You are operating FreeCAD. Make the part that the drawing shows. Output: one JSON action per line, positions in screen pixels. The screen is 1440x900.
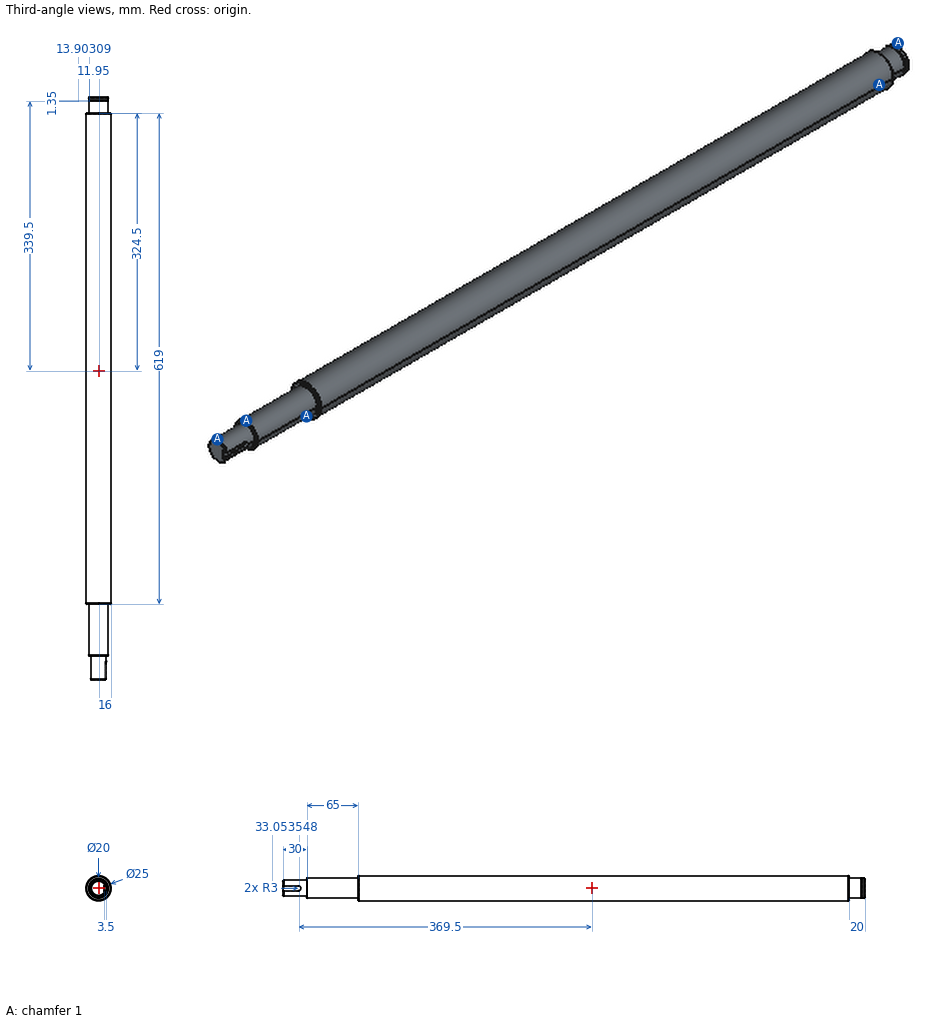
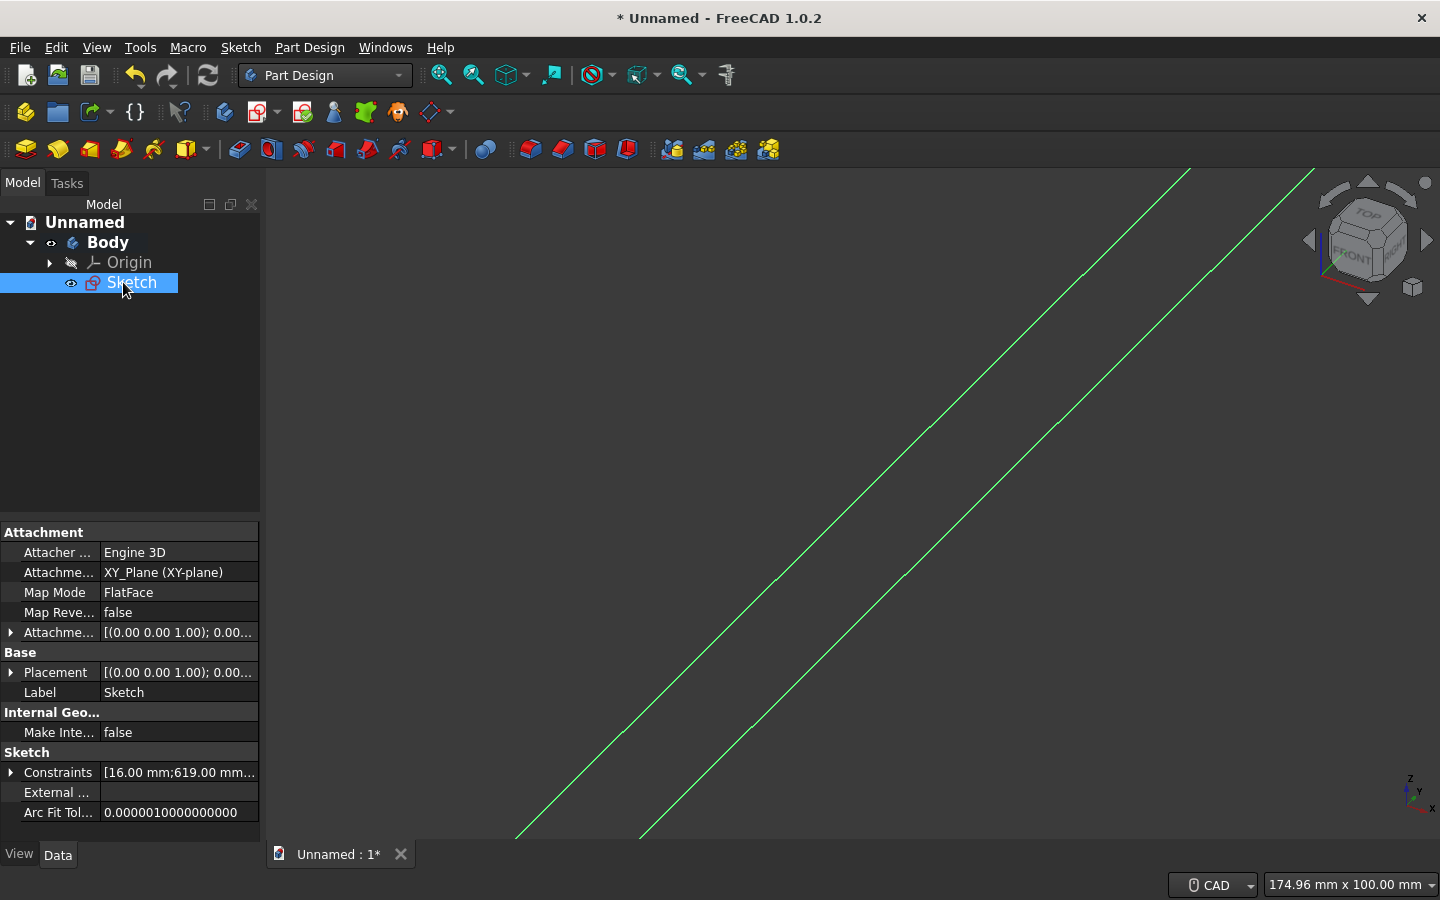
{"action": "left_click", "coordinate": [58, 150]}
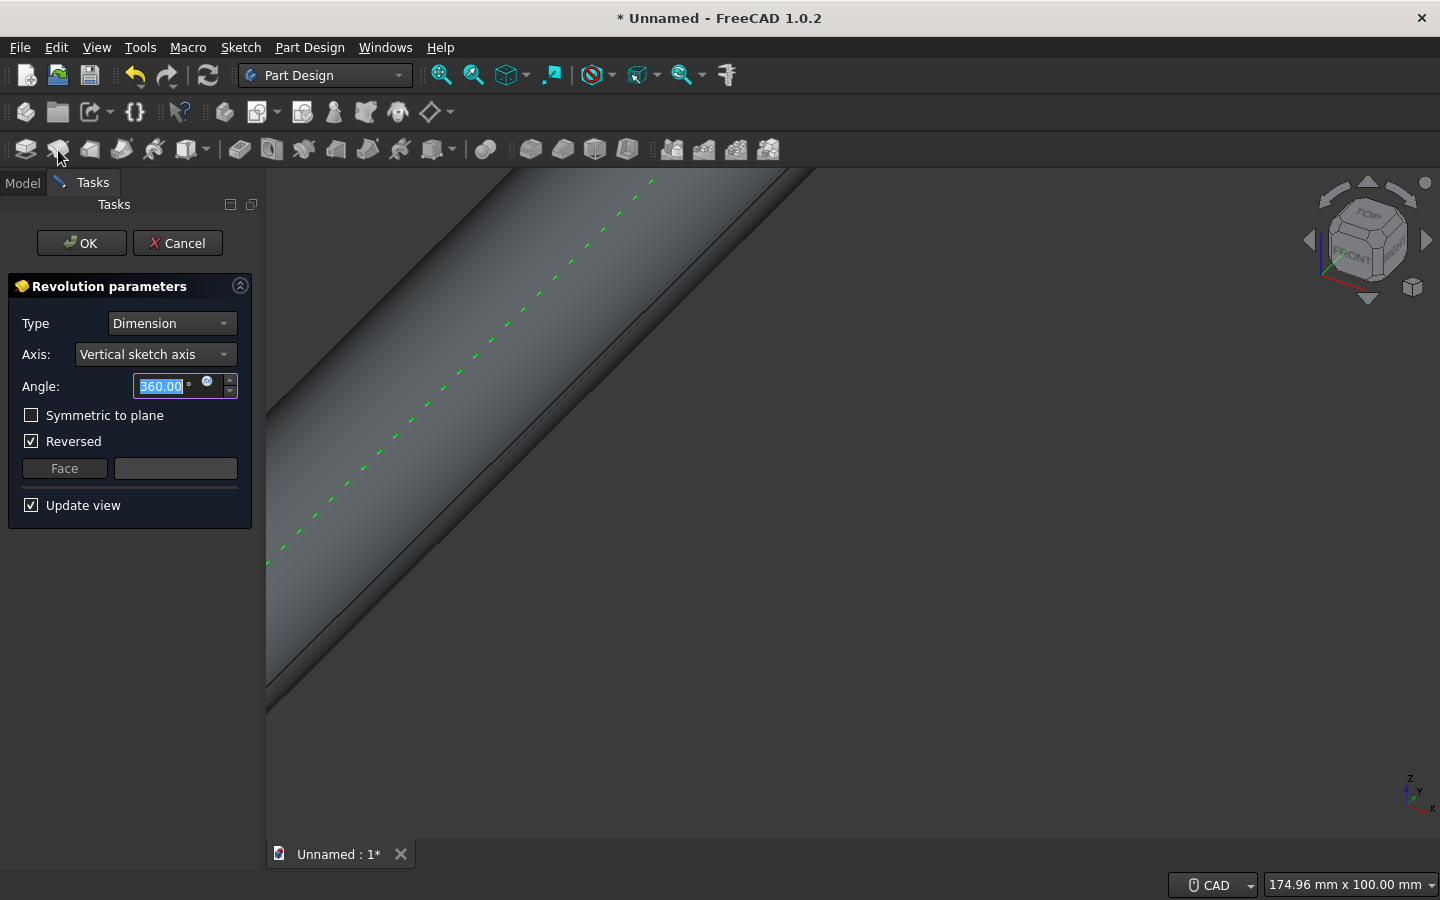
{"action": "left_click", "coordinate": [82, 243]}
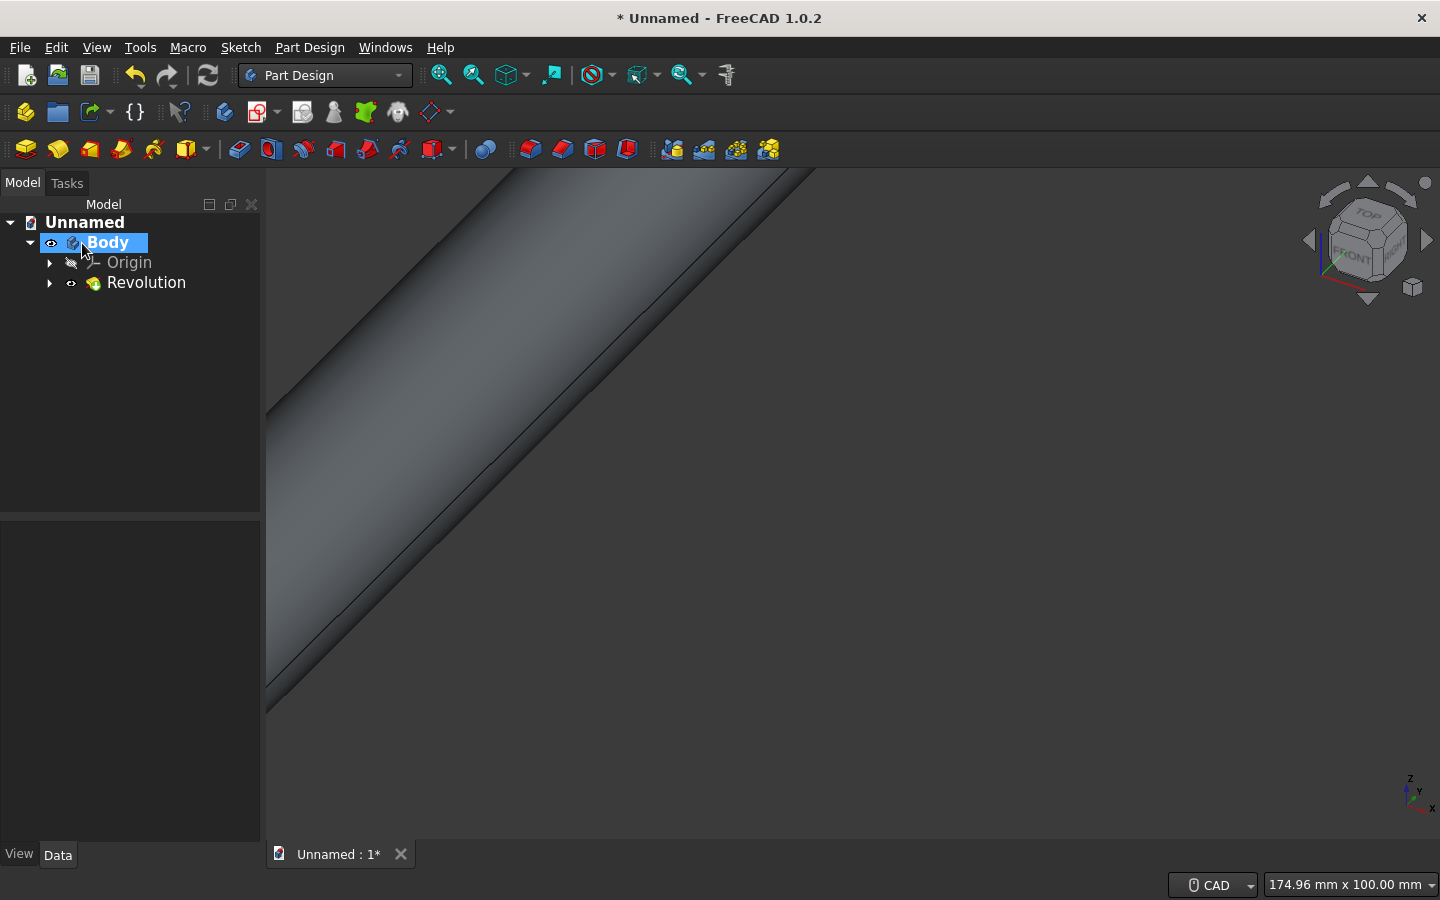
{"action": "left_click", "coordinate": [442, 76]}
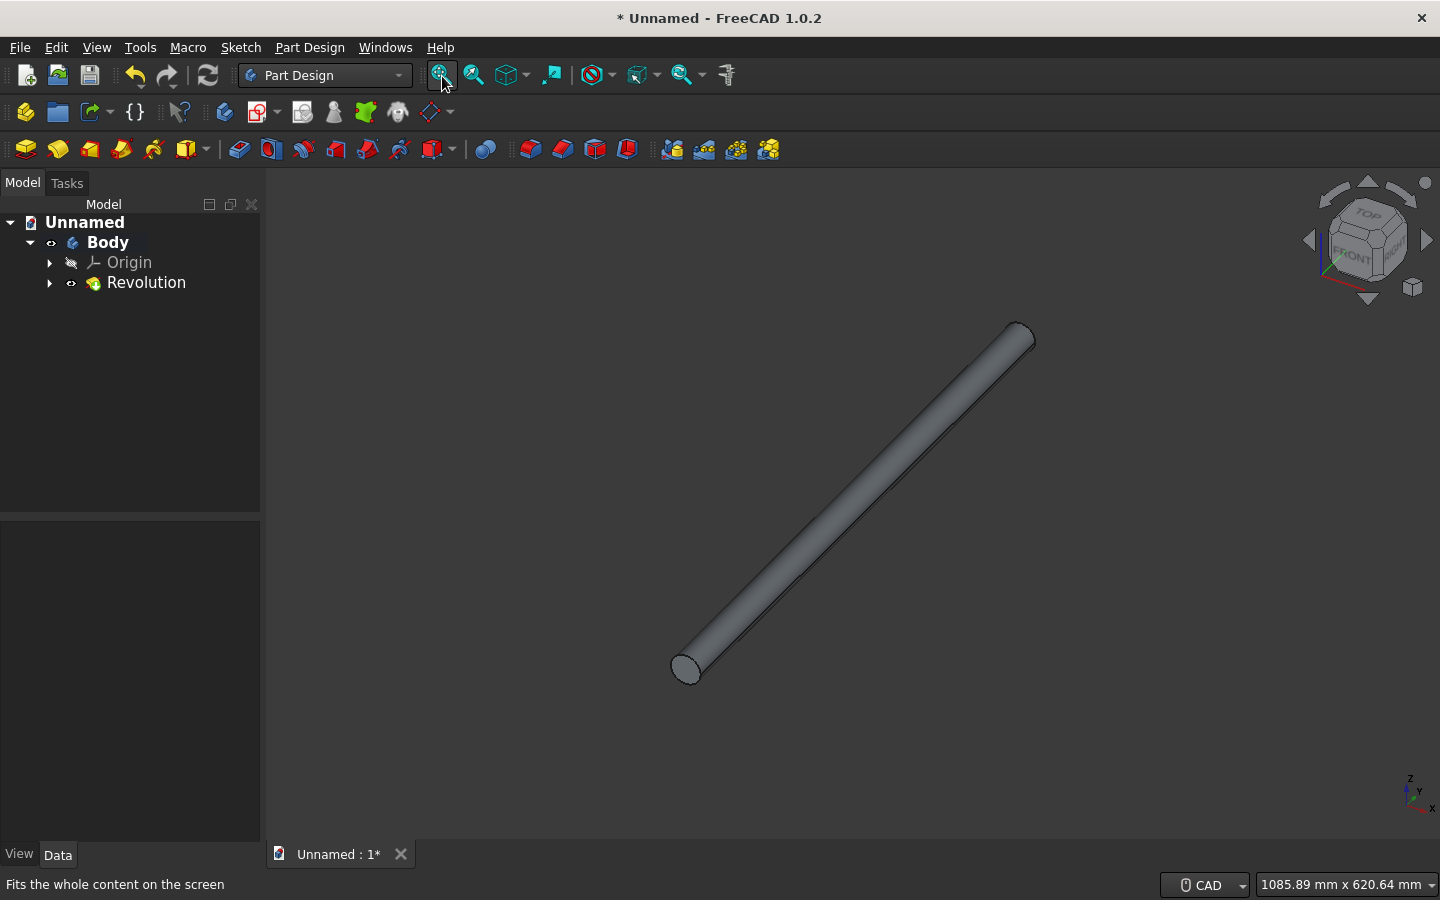
{"action": "left_click", "coordinate": [686, 669]}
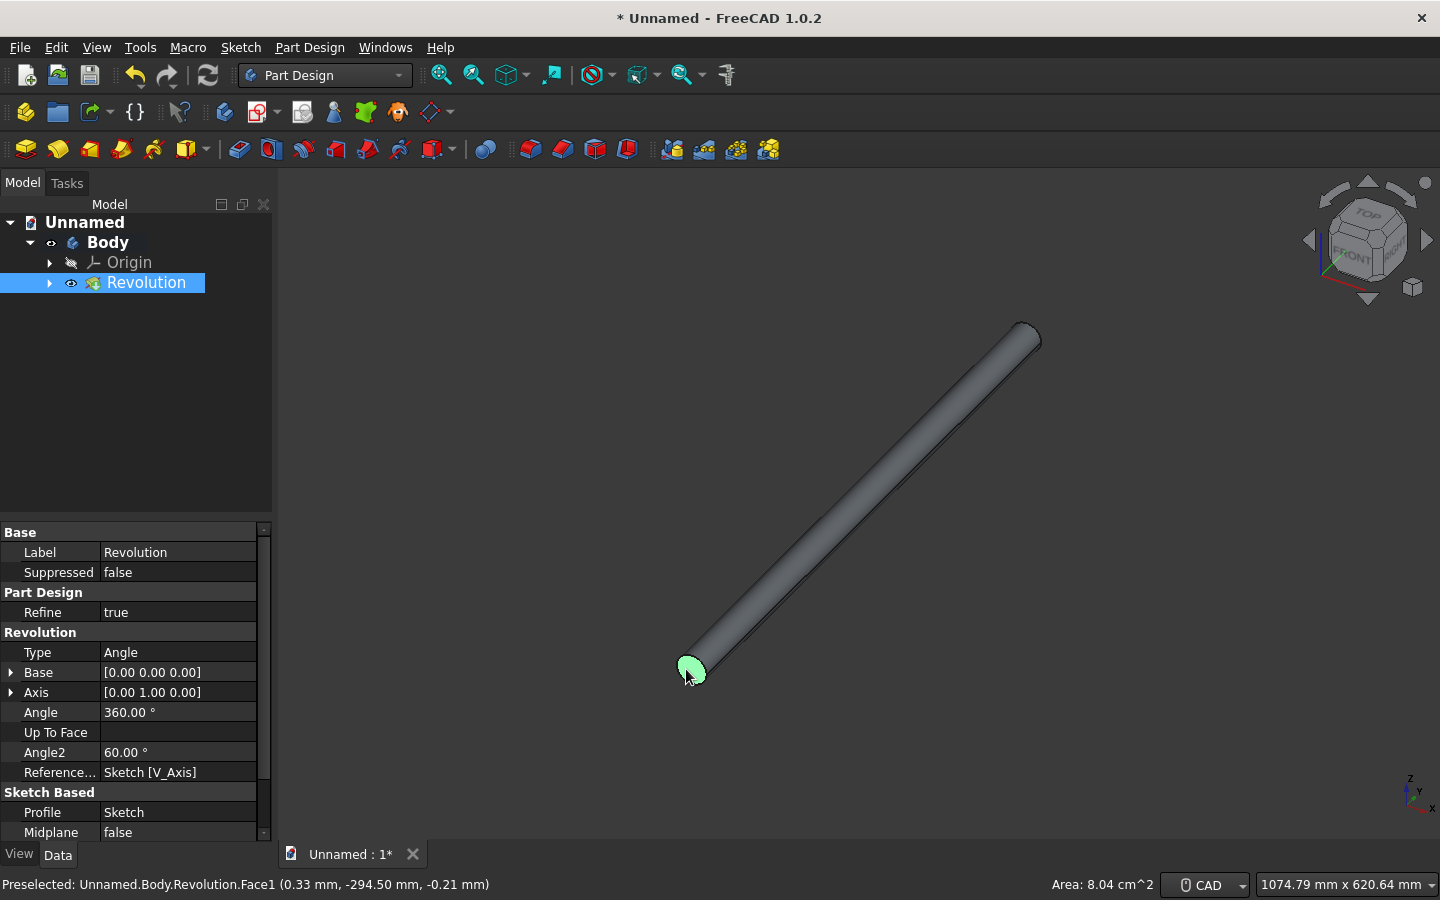
{"action": "left_click", "coordinate": [258, 112]}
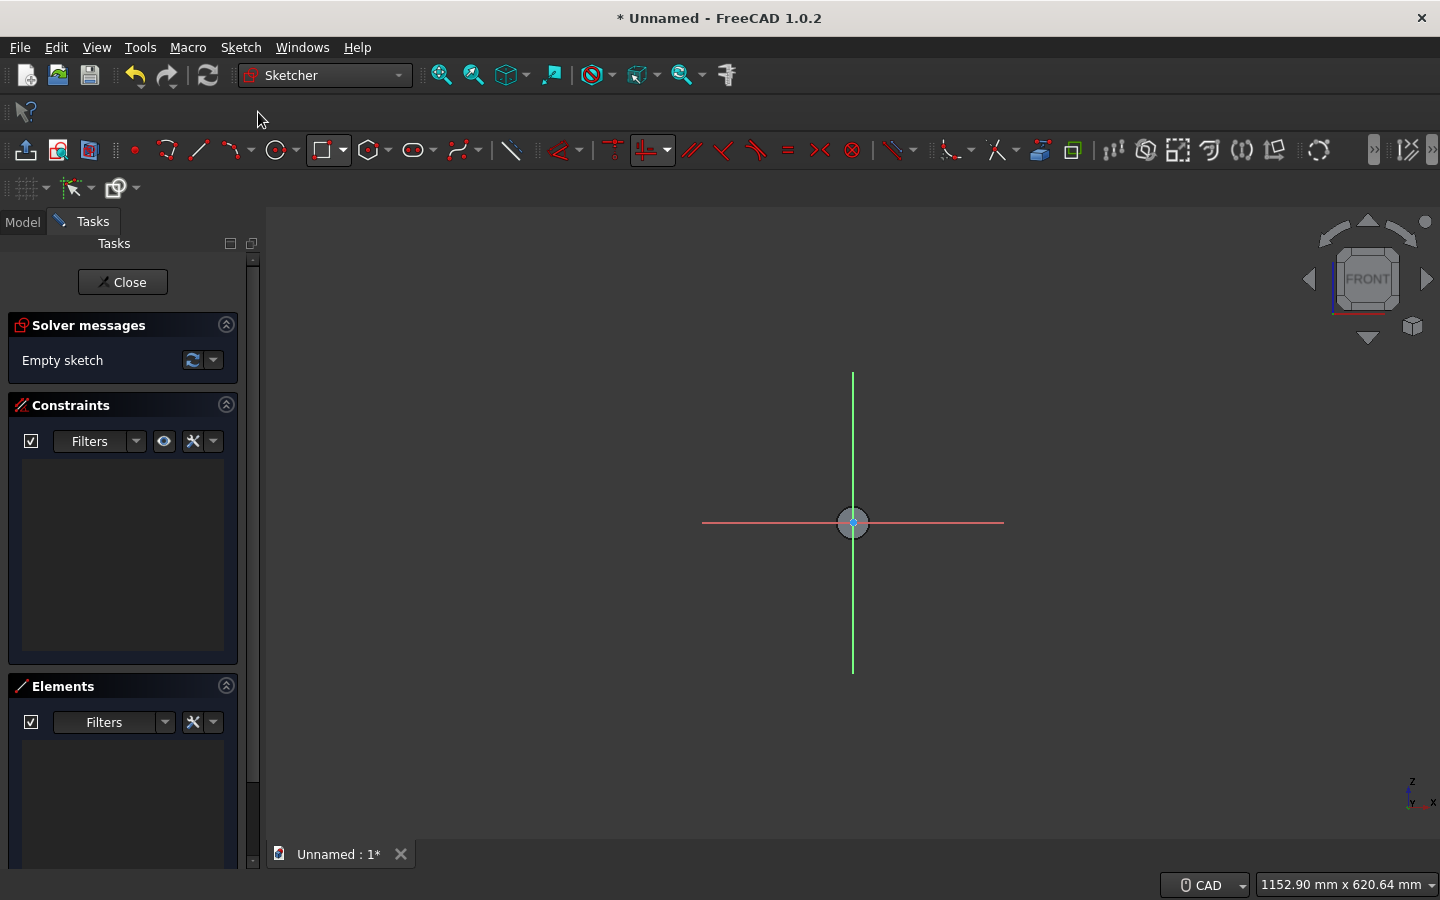
{"action": "scroll", "coordinate": [857, 523], "scroll_direction": "up", "scroll_amount": 14}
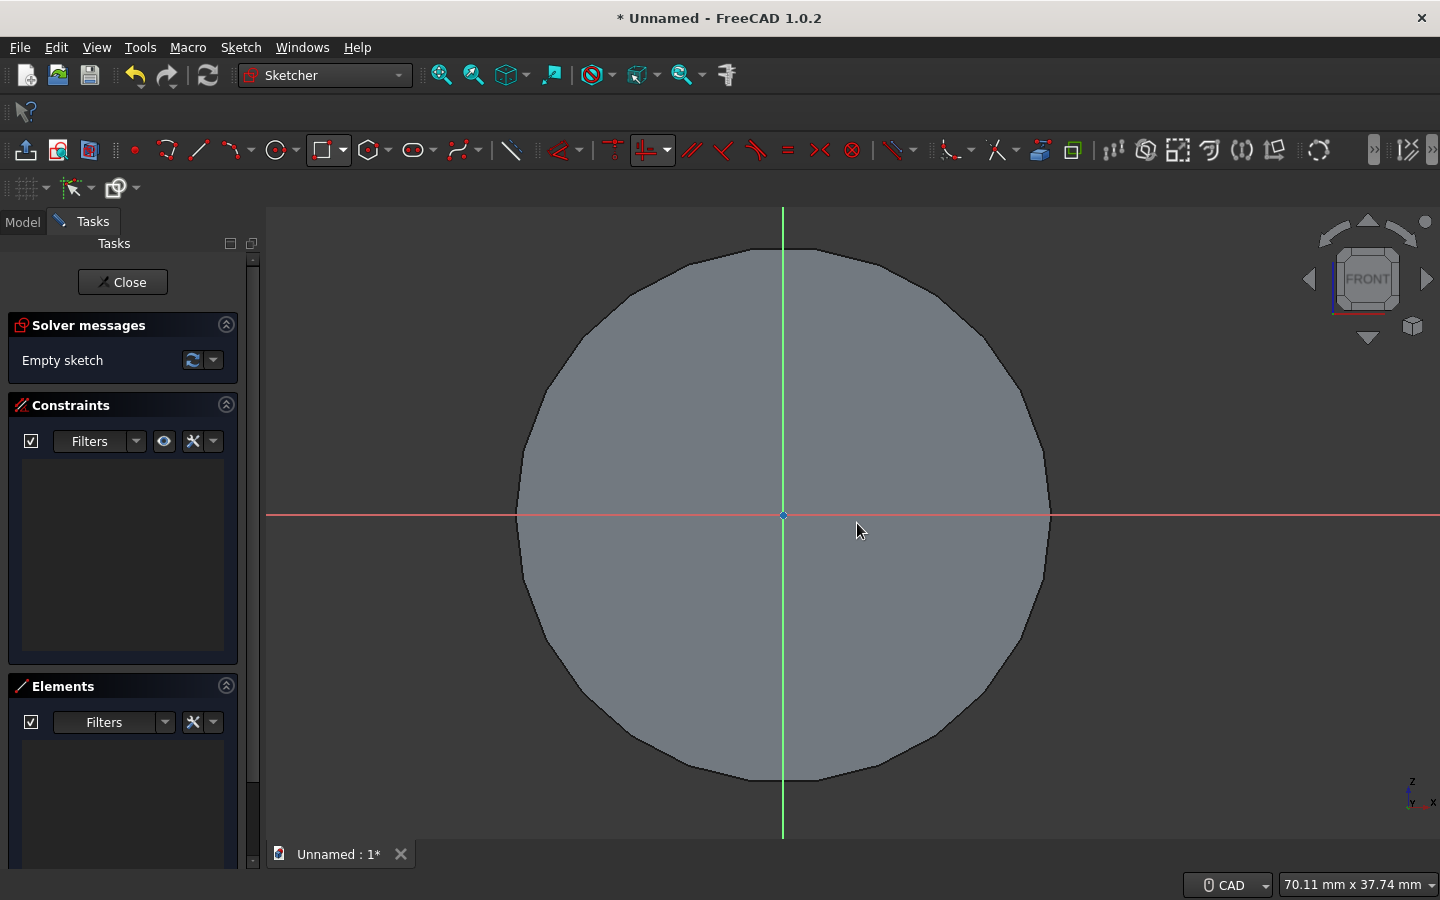
{"action": "left_click", "coordinate": [276, 150]}